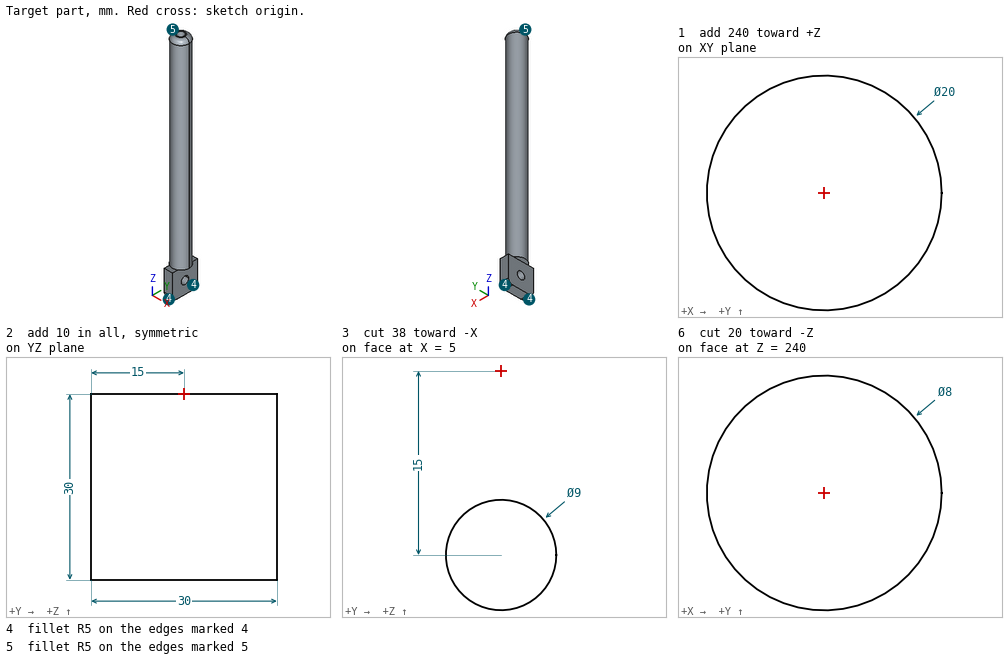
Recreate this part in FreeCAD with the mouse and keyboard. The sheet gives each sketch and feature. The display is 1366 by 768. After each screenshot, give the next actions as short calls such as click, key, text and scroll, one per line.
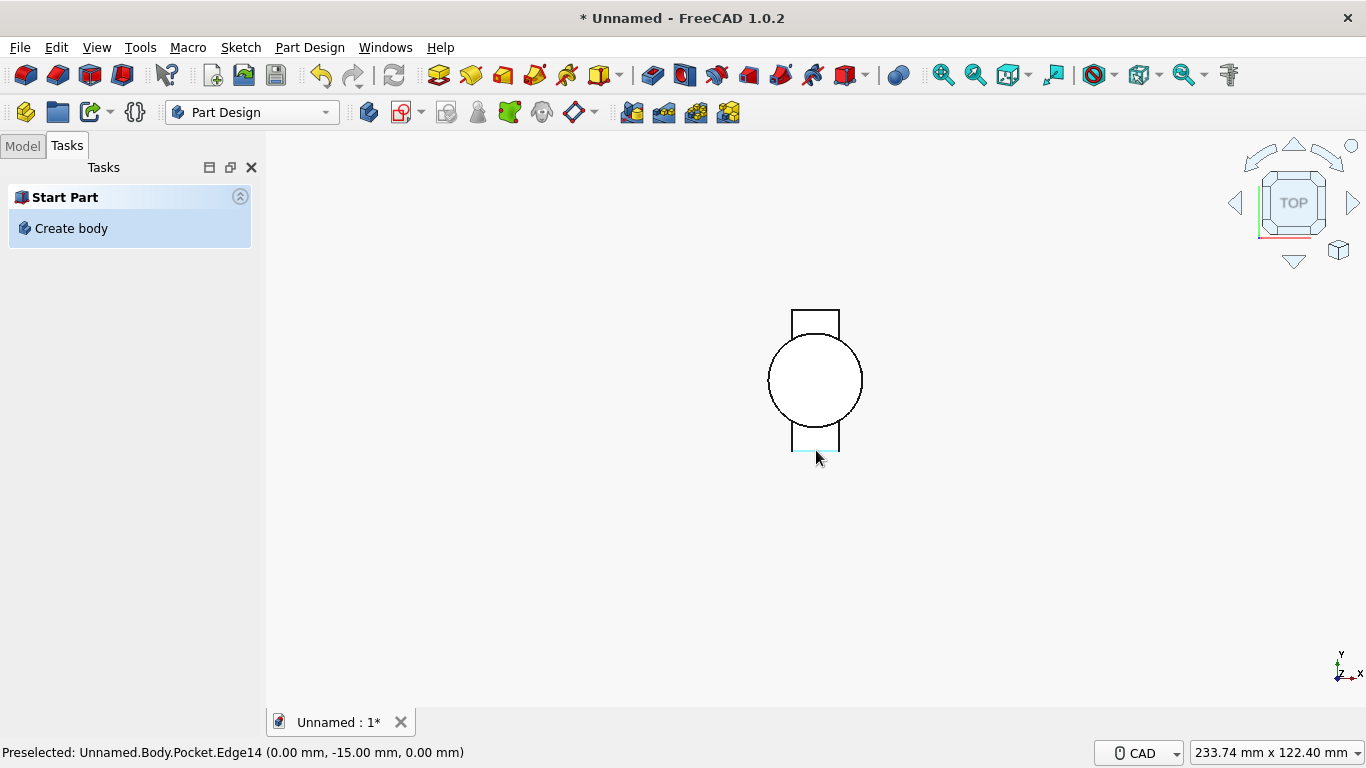
key(v)
key(f)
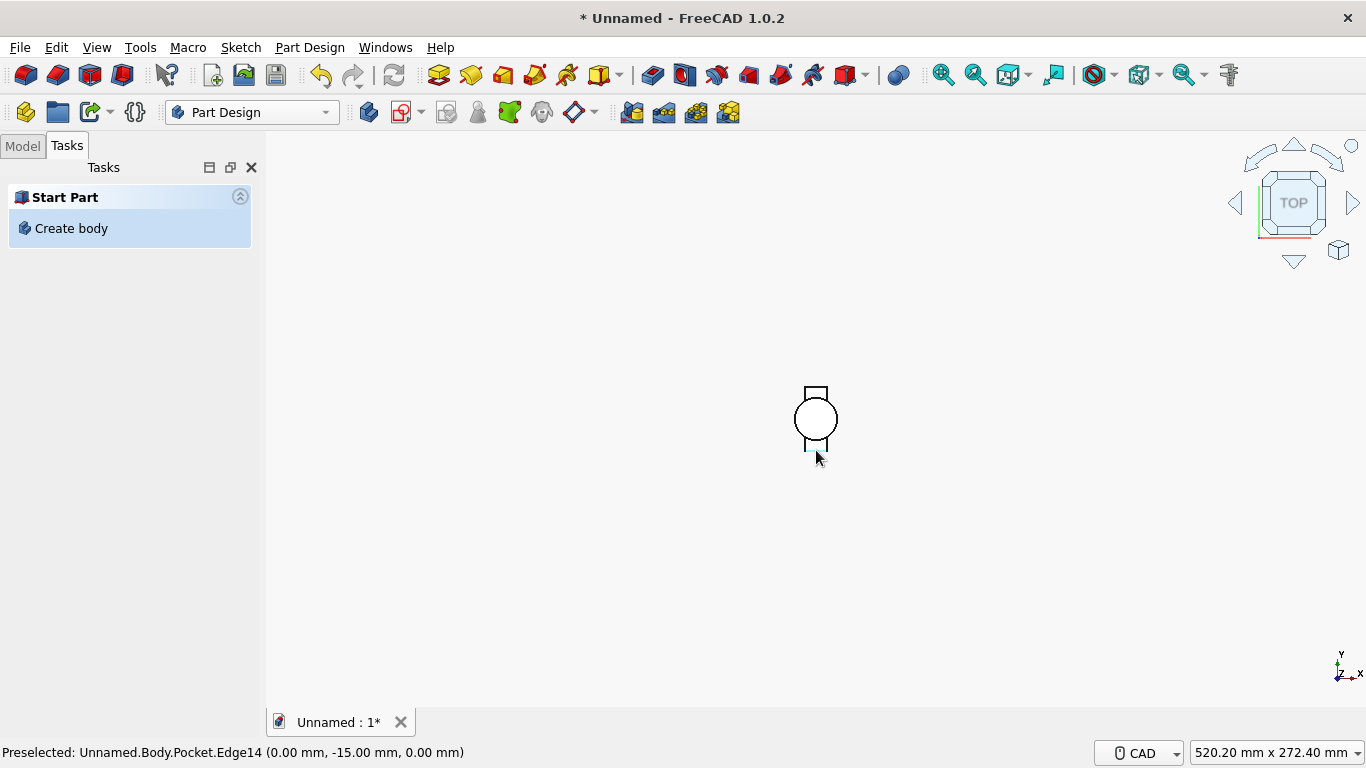
key(1)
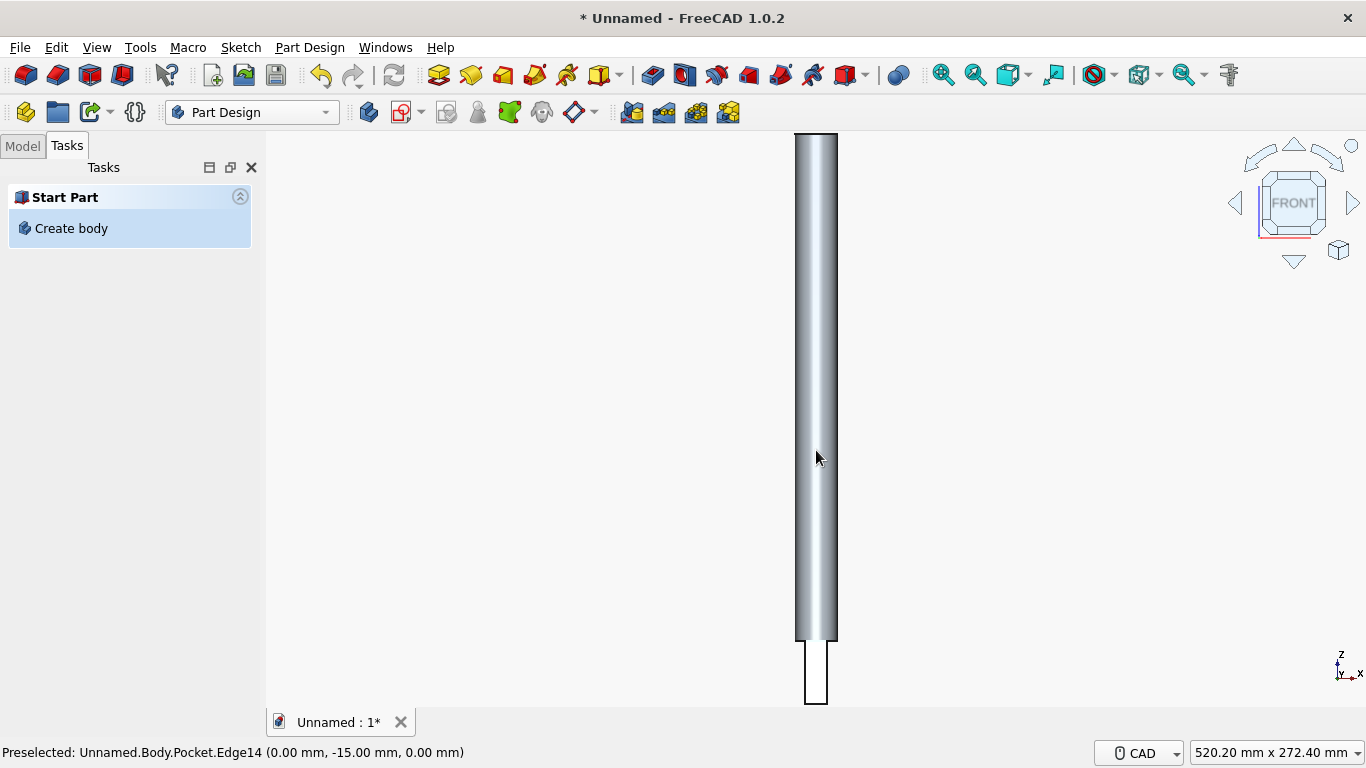
key(3)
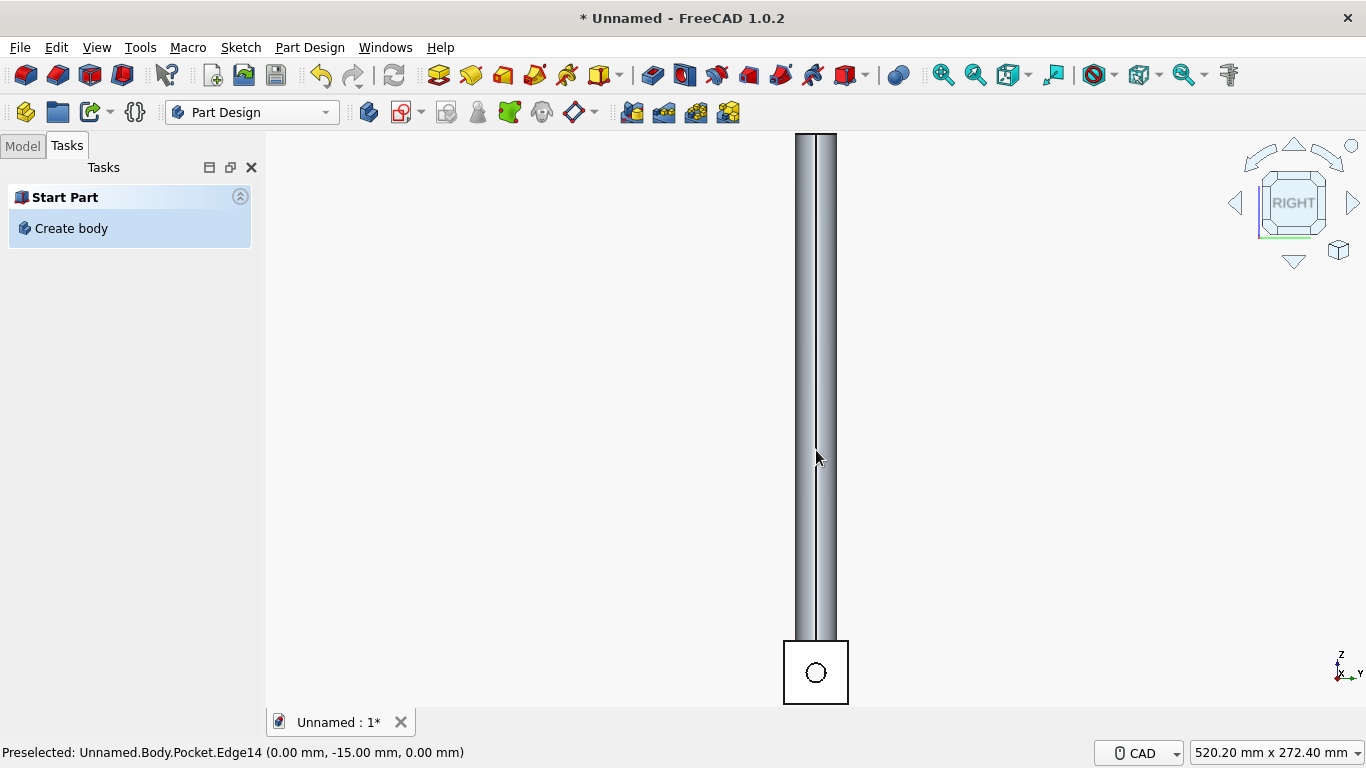
key(5)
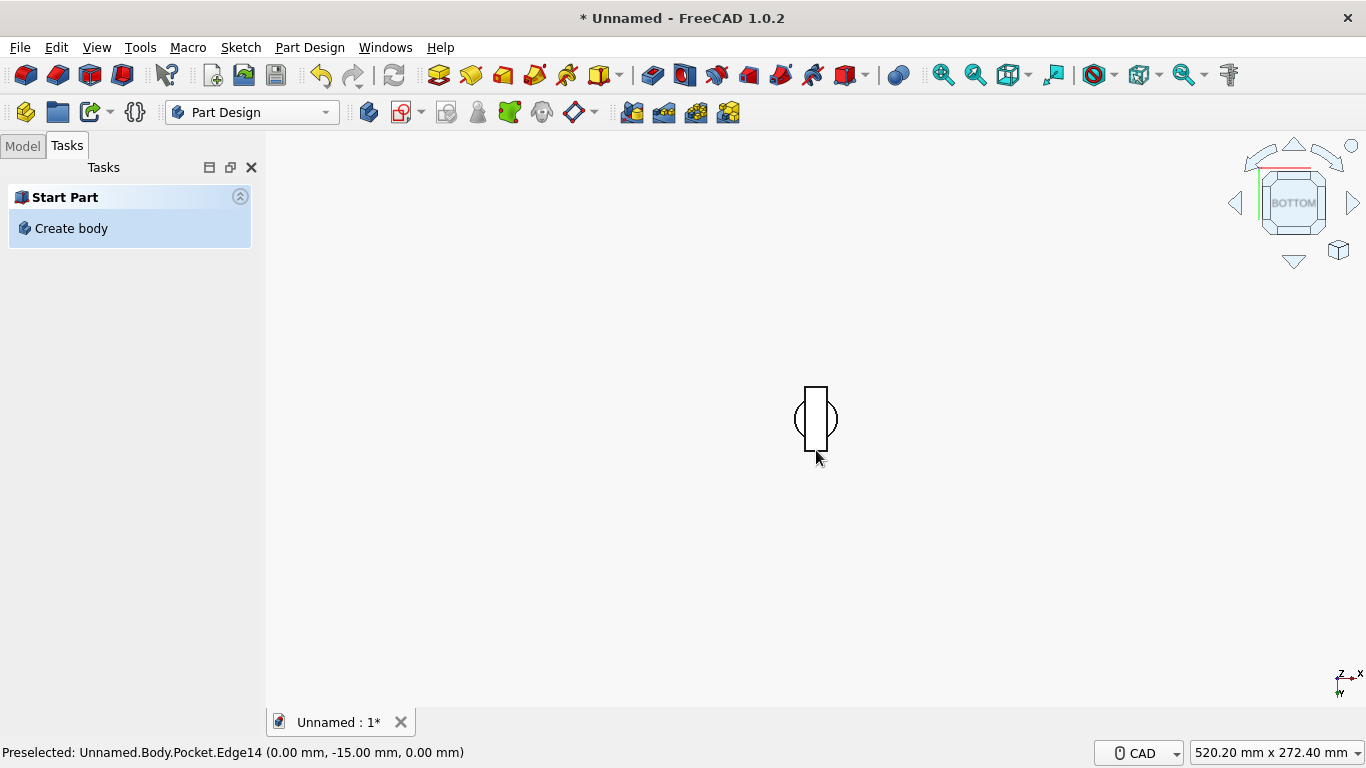
key(v)
key(f)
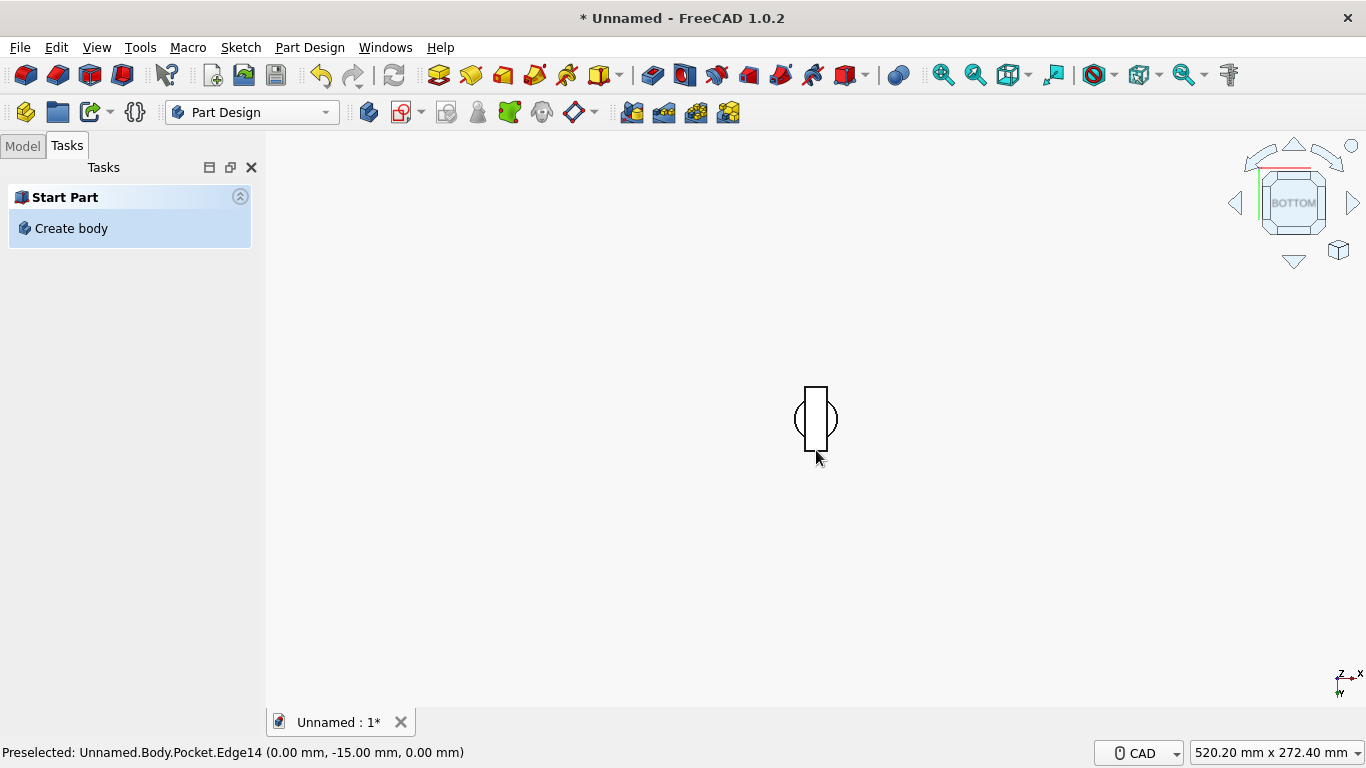
click(816, 386)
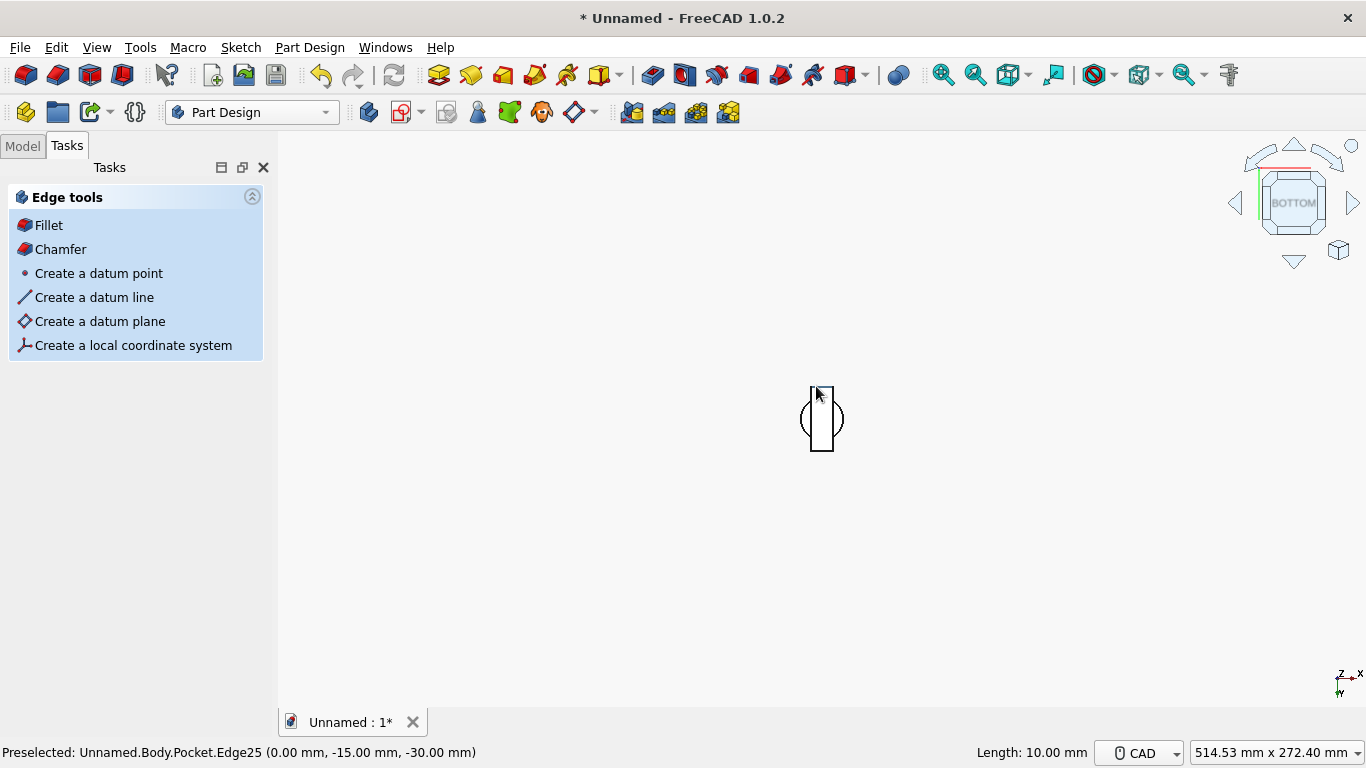
click(822, 450, ctrl)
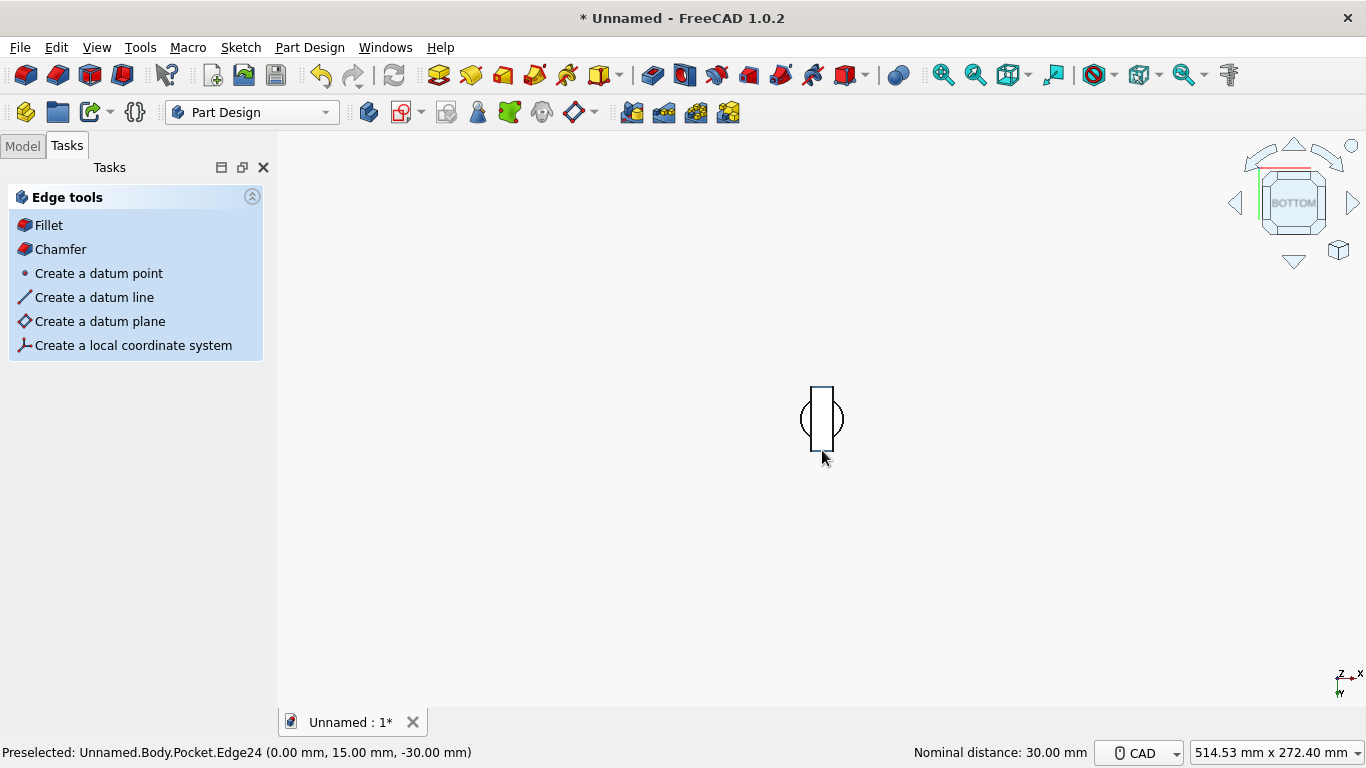
click(26, 76)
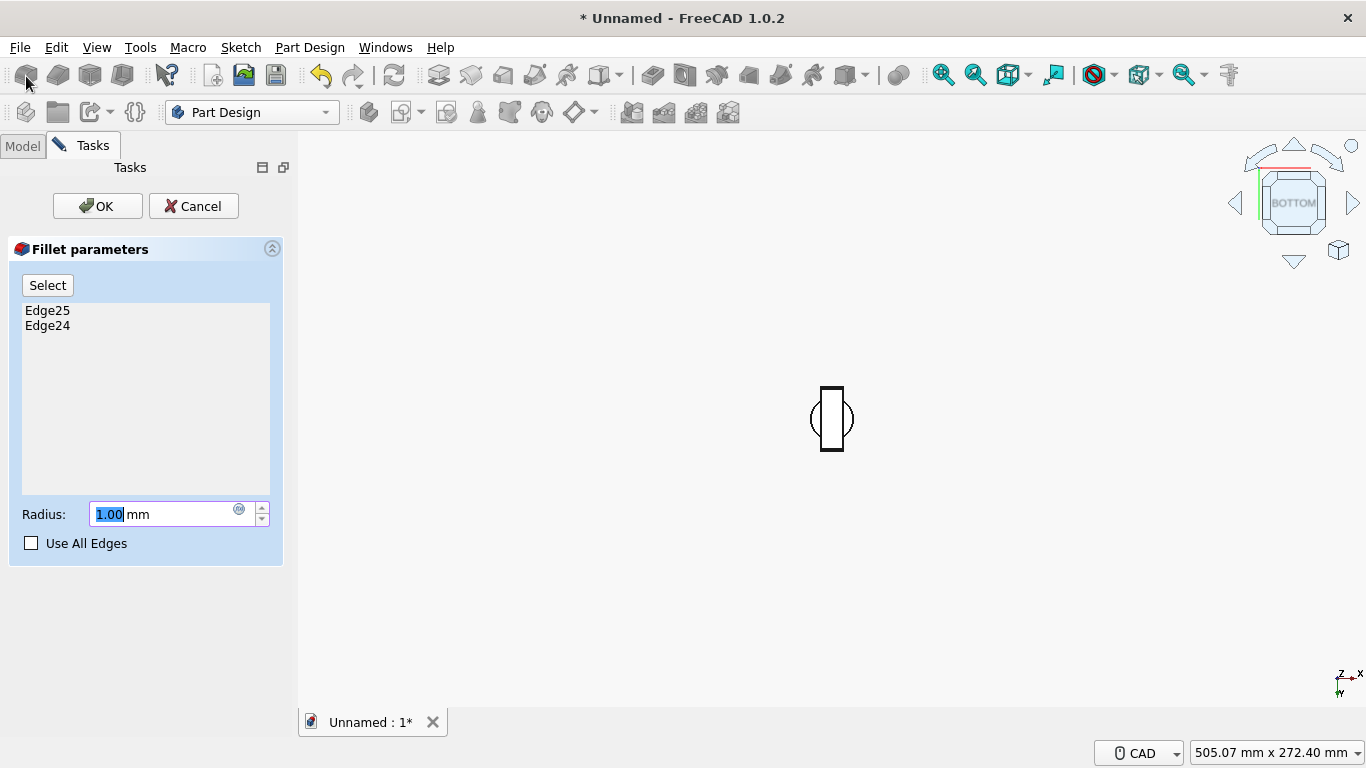
text(5)
key(Tab)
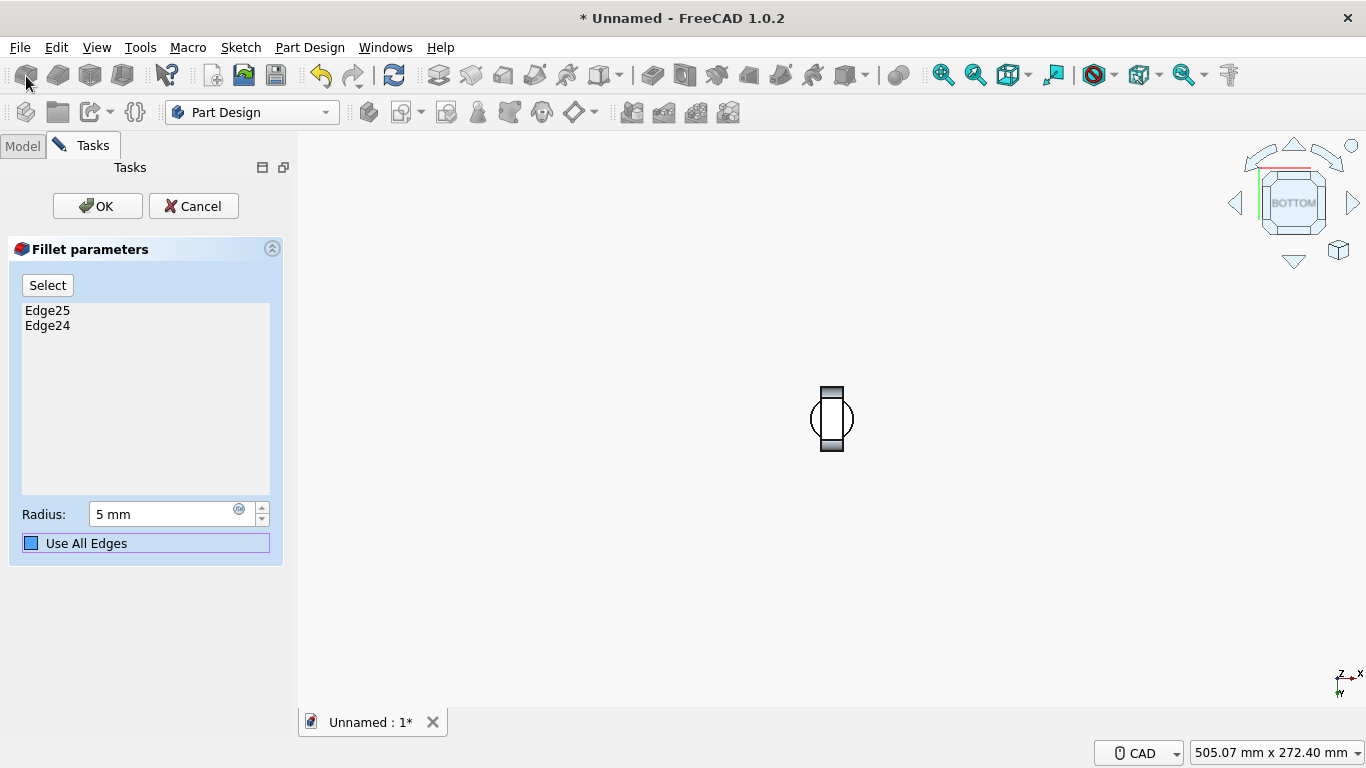
click(98, 206)